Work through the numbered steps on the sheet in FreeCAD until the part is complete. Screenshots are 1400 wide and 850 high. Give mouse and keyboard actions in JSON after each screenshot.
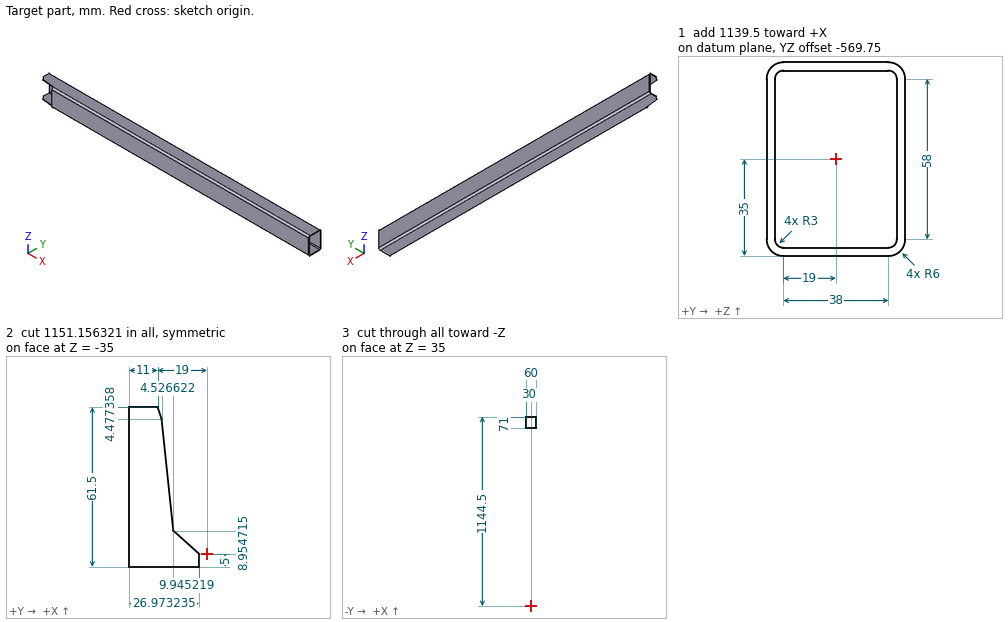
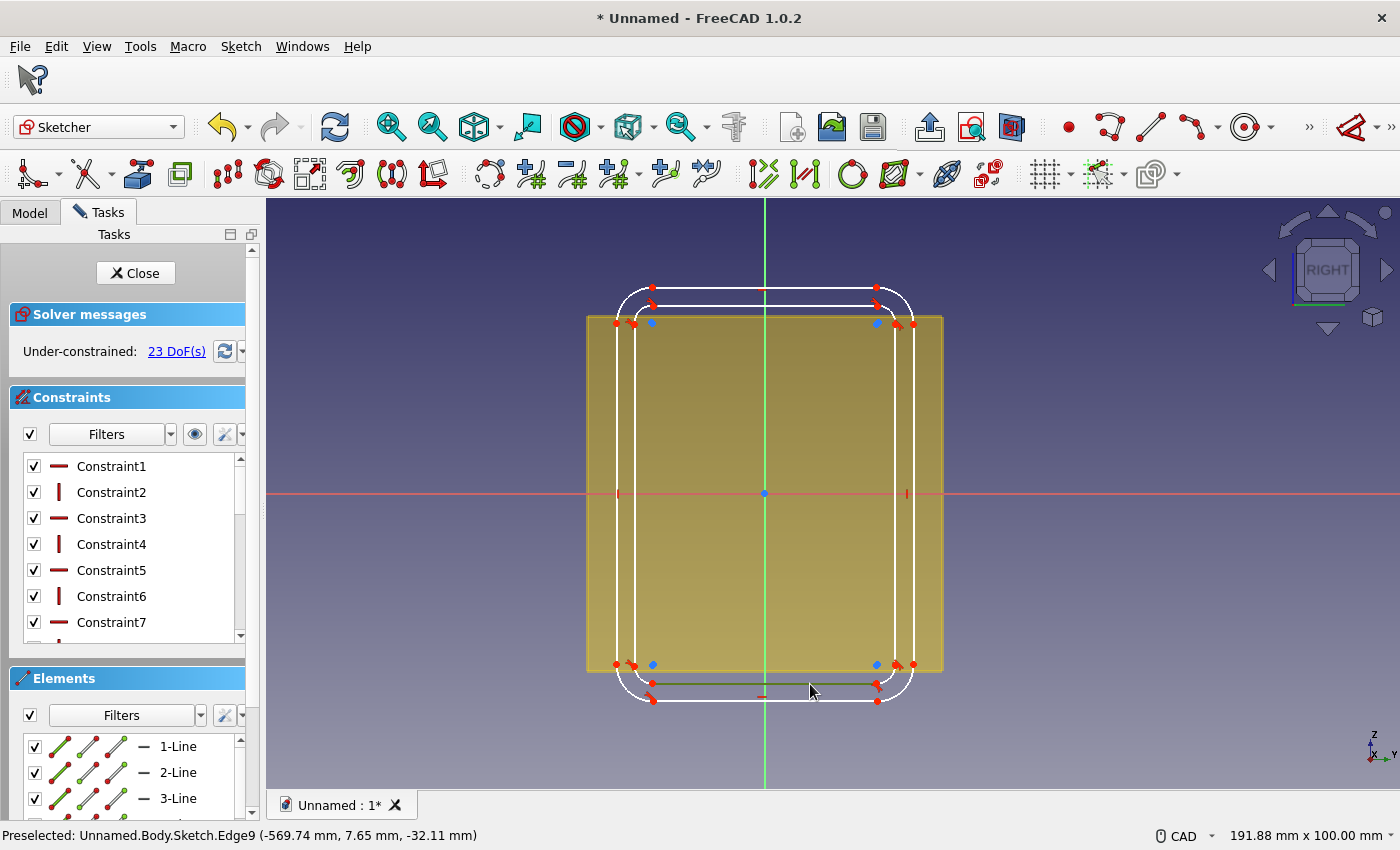
{"action": "left_click", "coordinate": [890, 679]}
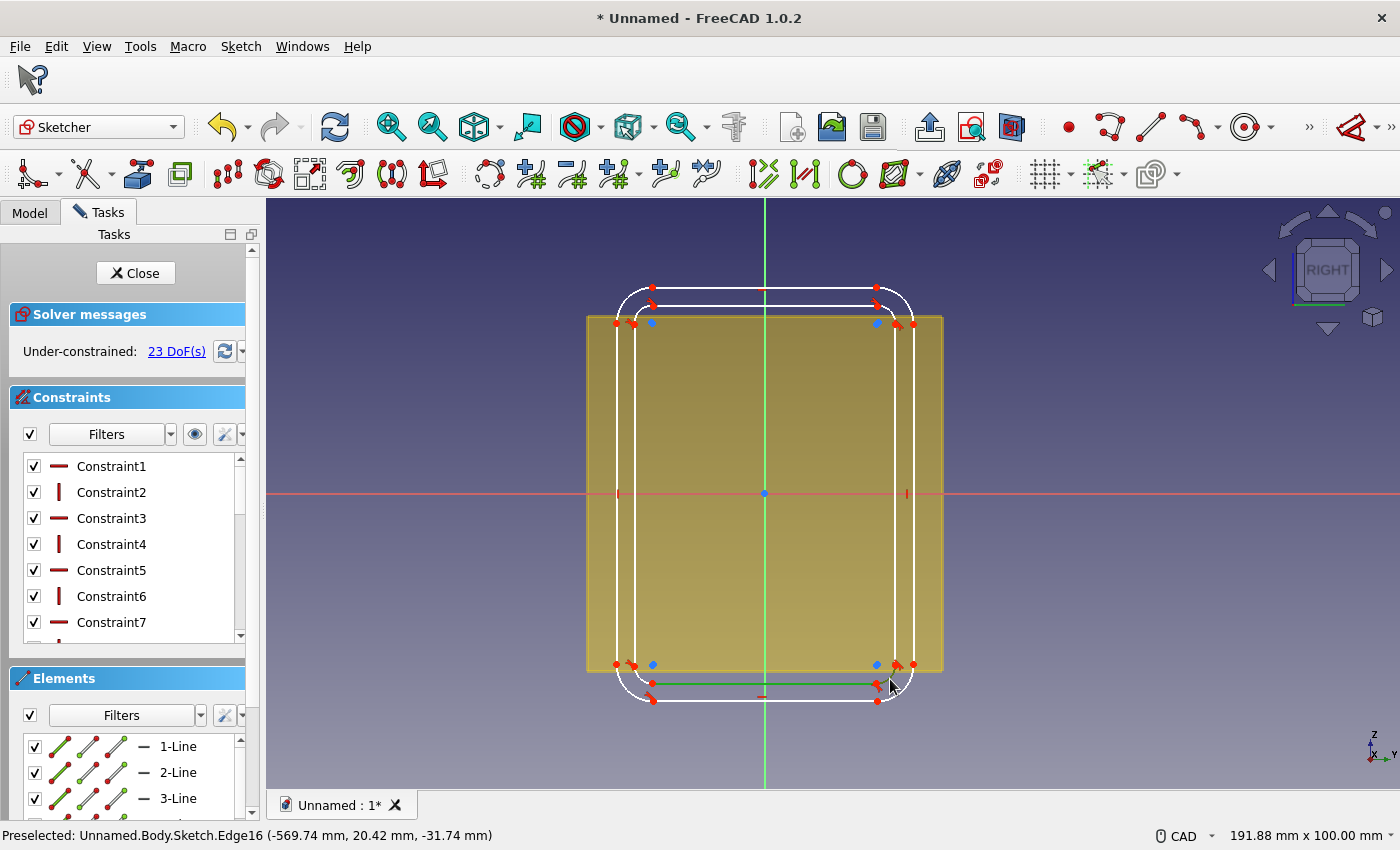
{"action": "key", "text": "t"}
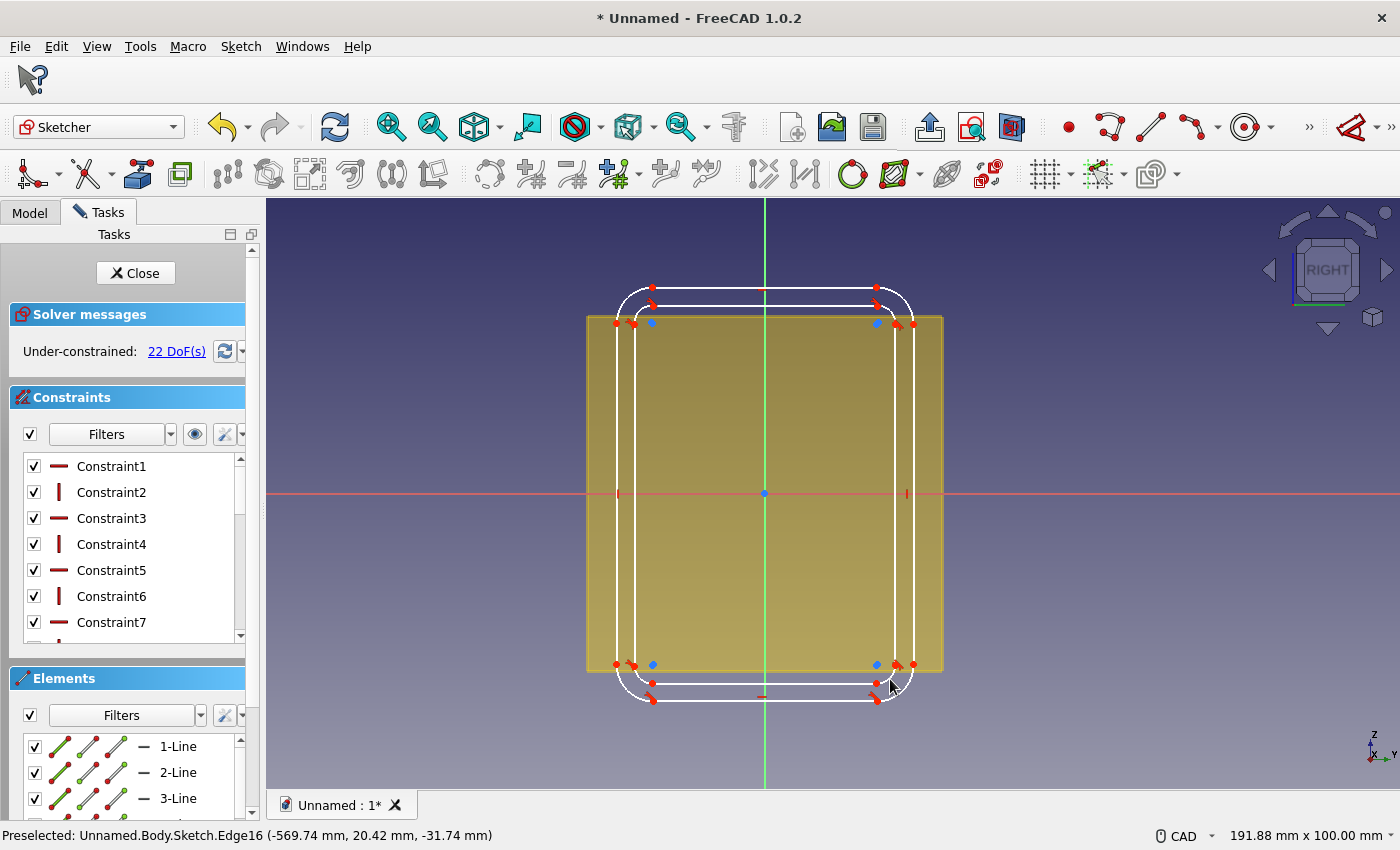
{"action": "left_click", "coordinate": [635, 563]}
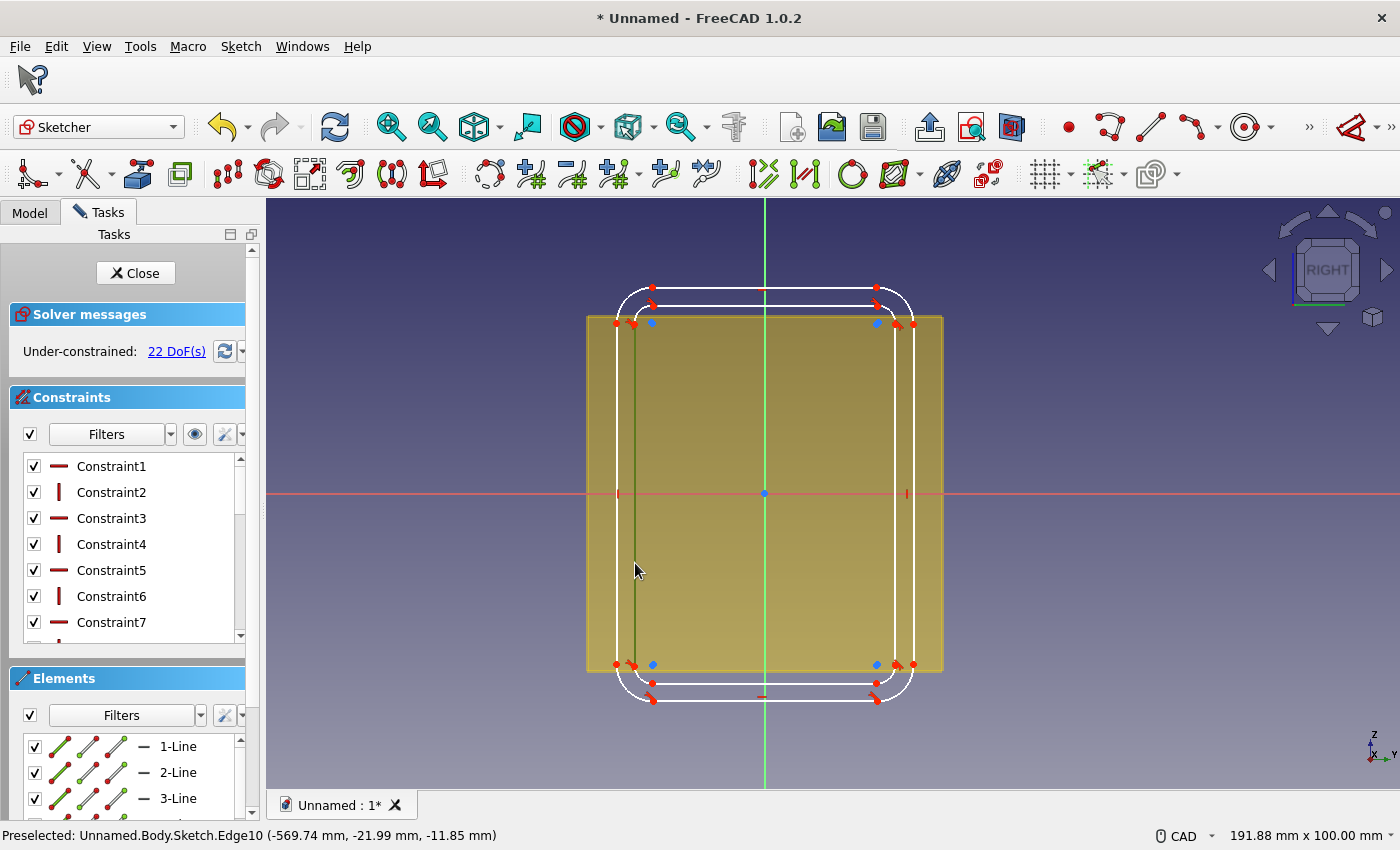
{"action": "left_click", "coordinate": [640, 679]}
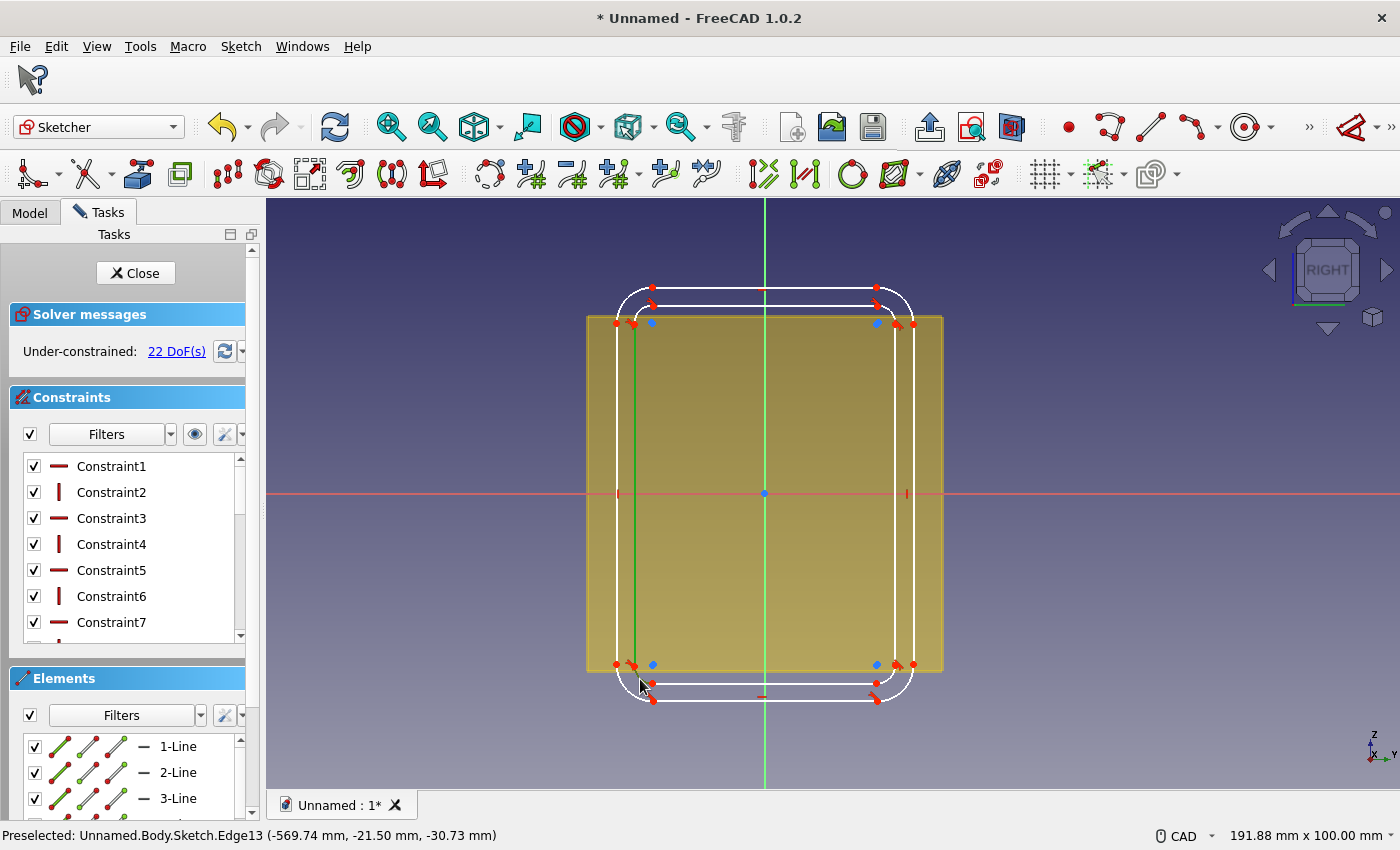
{"action": "key", "text": "t"}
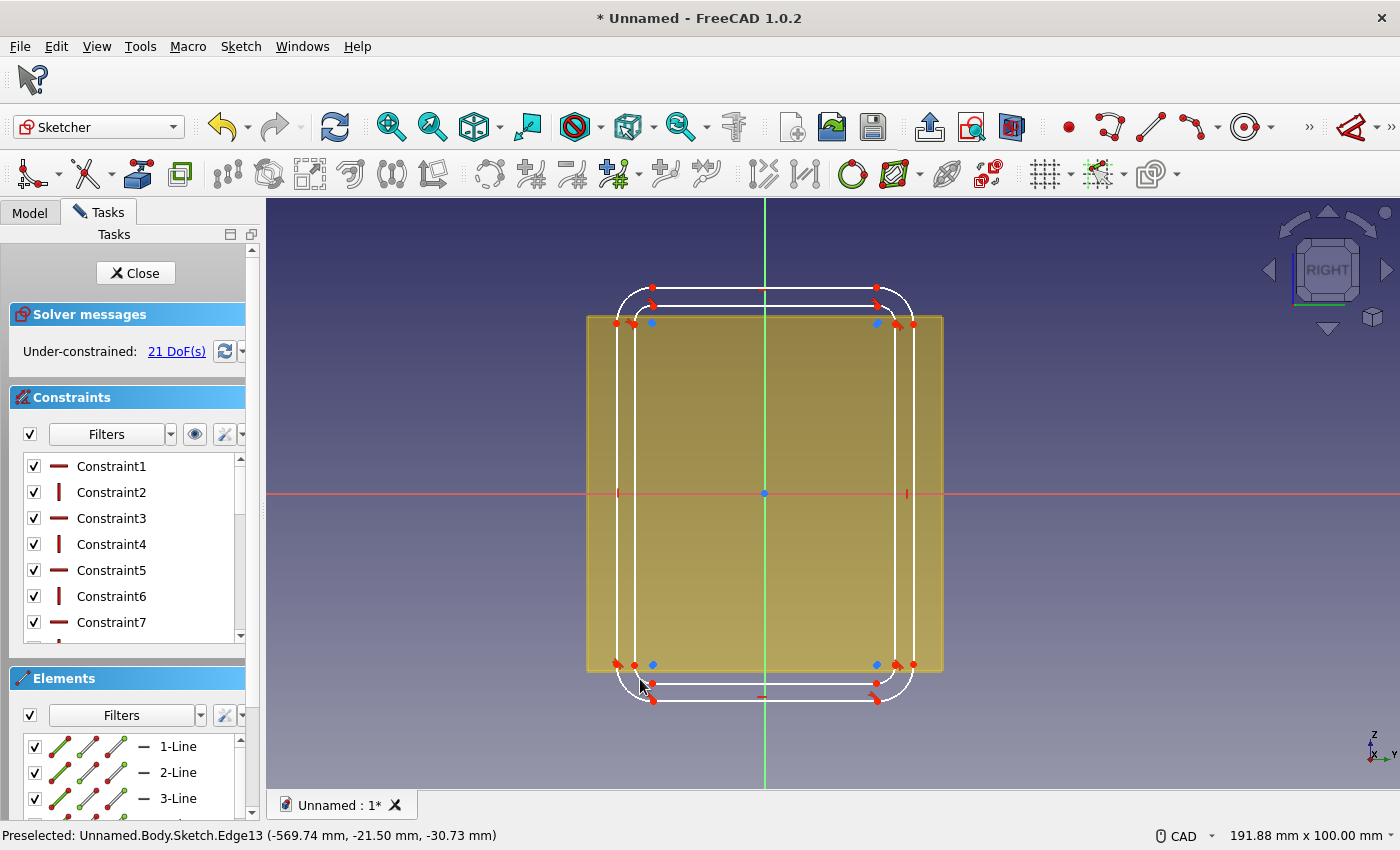
{"action": "left_click", "coordinate": [635, 563]}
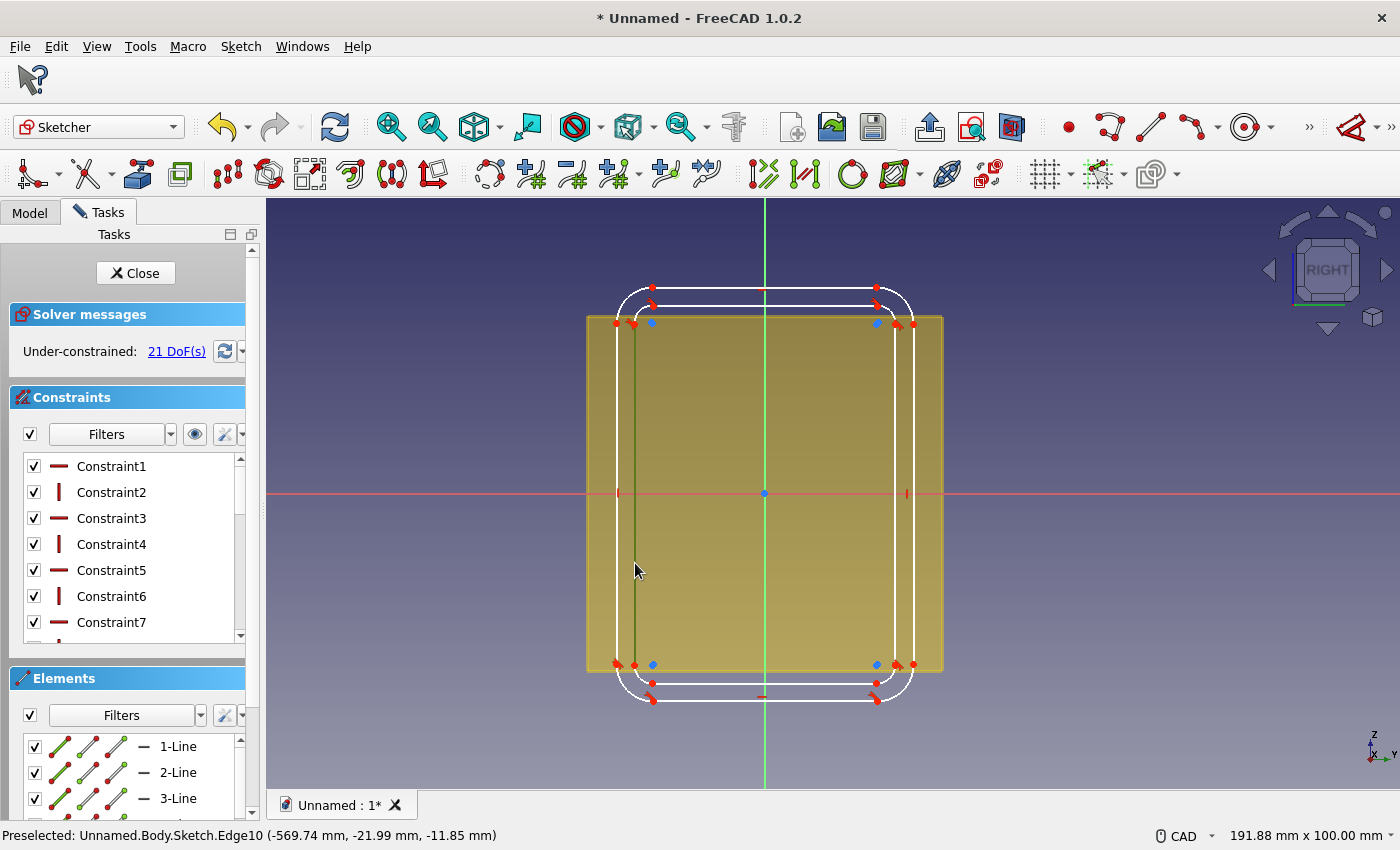
{"action": "left_click", "coordinate": [640, 311]}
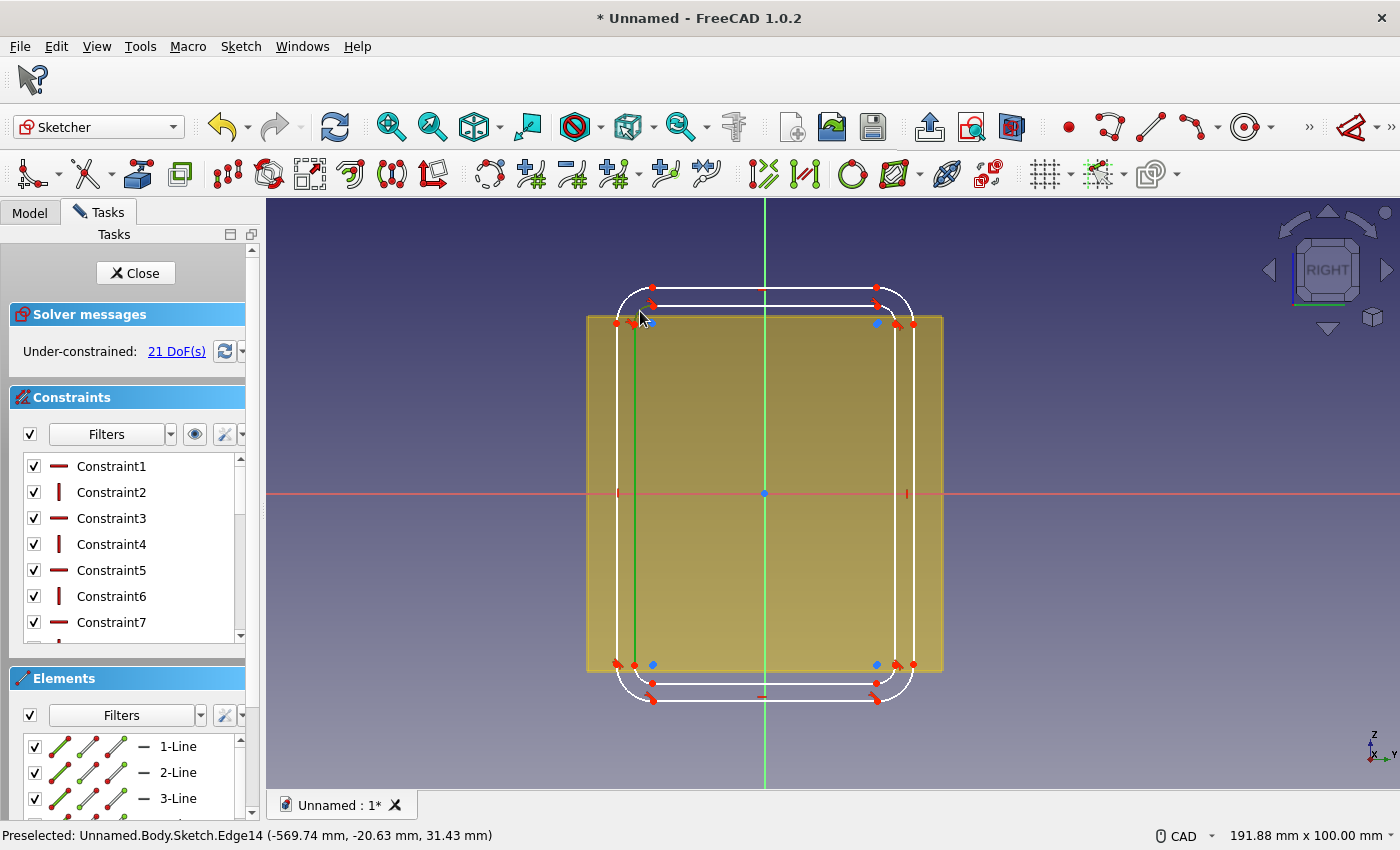
{"action": "key", "text": "t"}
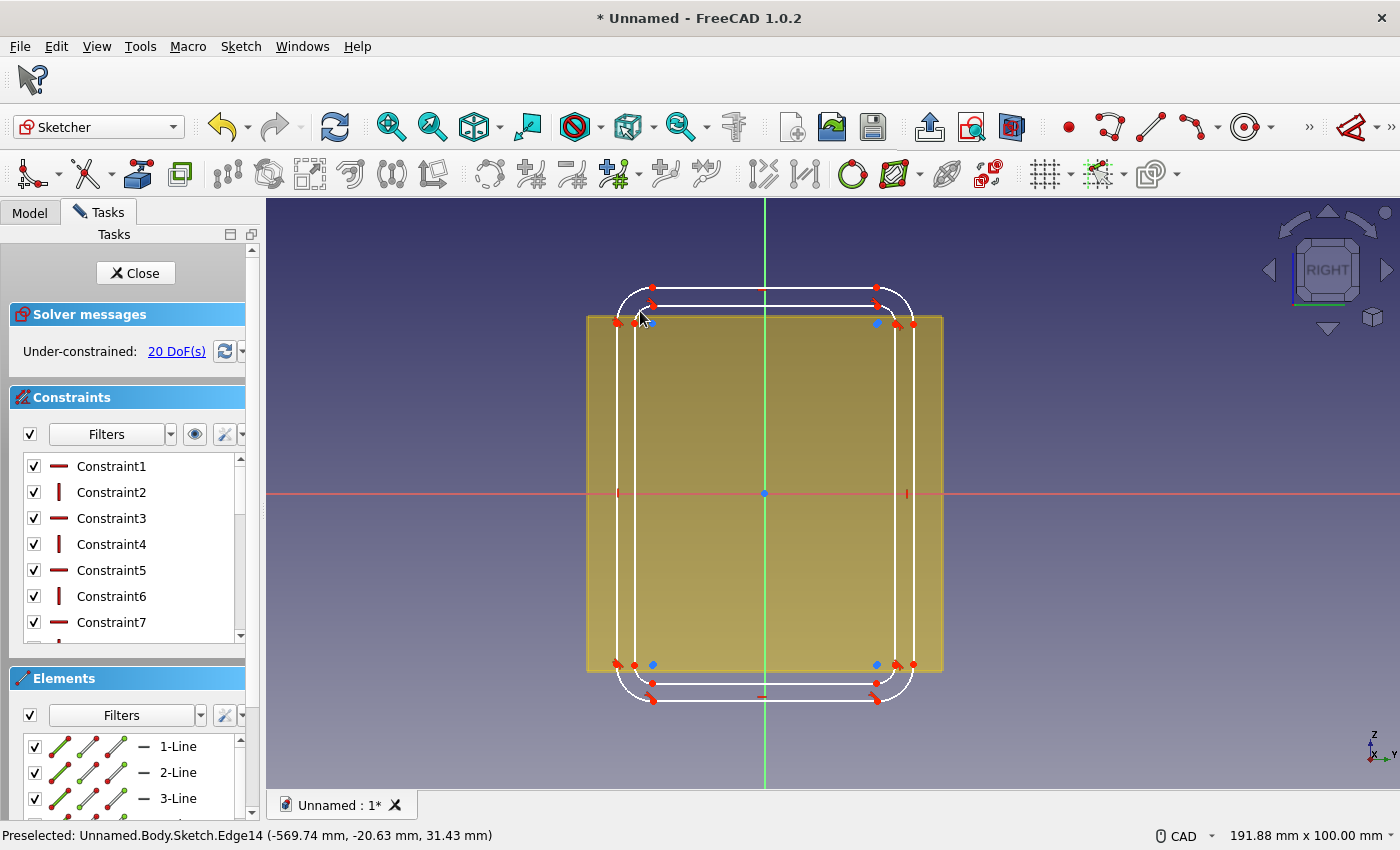
{"action": "left_click", "coordinate": [720, 306]}